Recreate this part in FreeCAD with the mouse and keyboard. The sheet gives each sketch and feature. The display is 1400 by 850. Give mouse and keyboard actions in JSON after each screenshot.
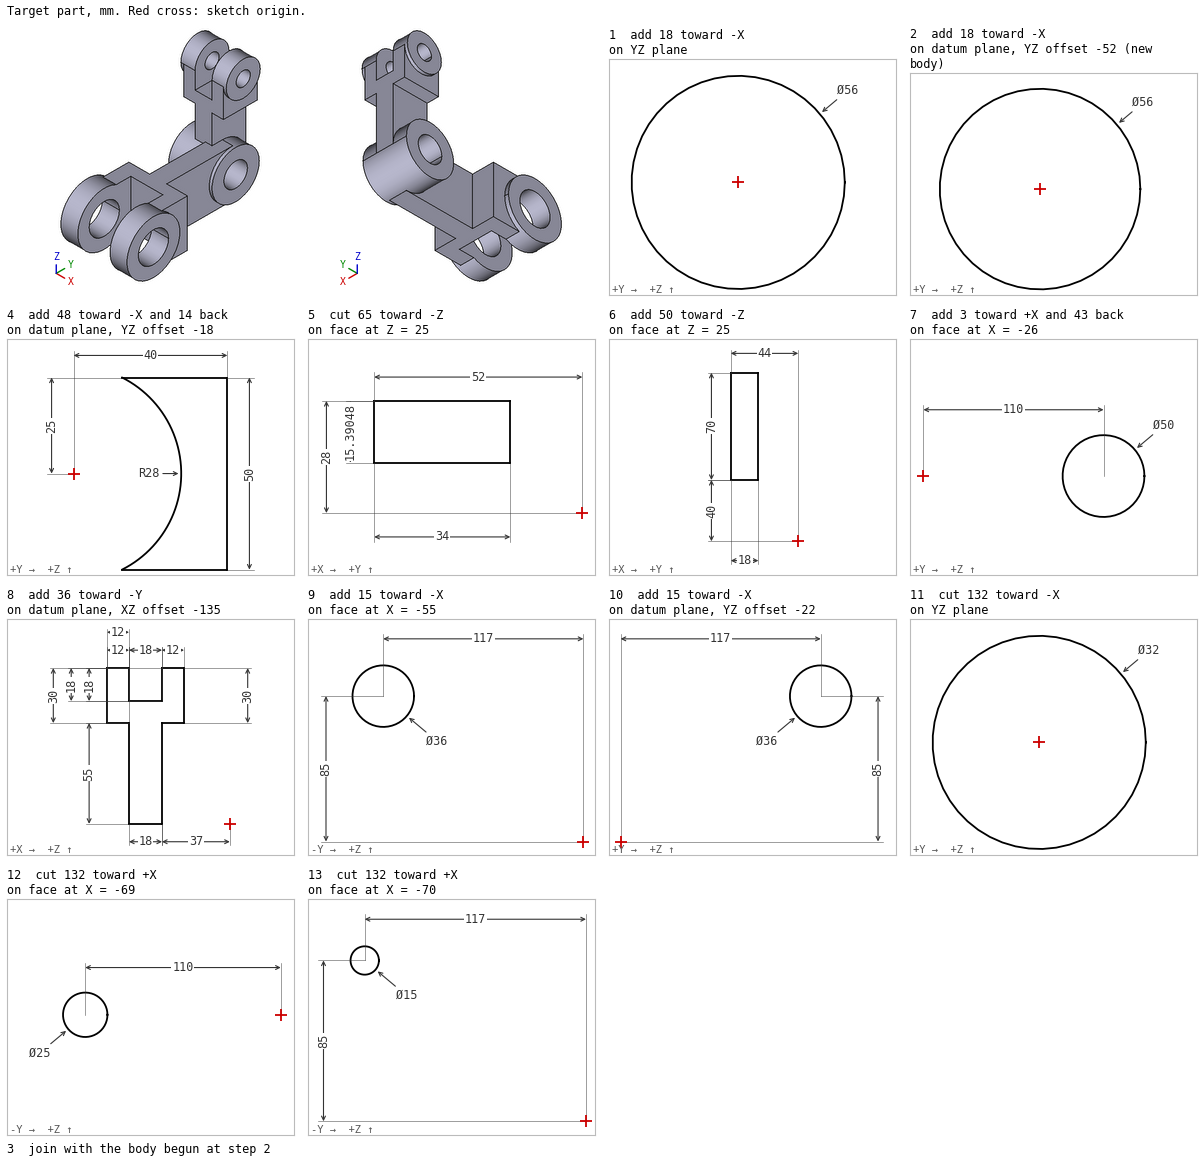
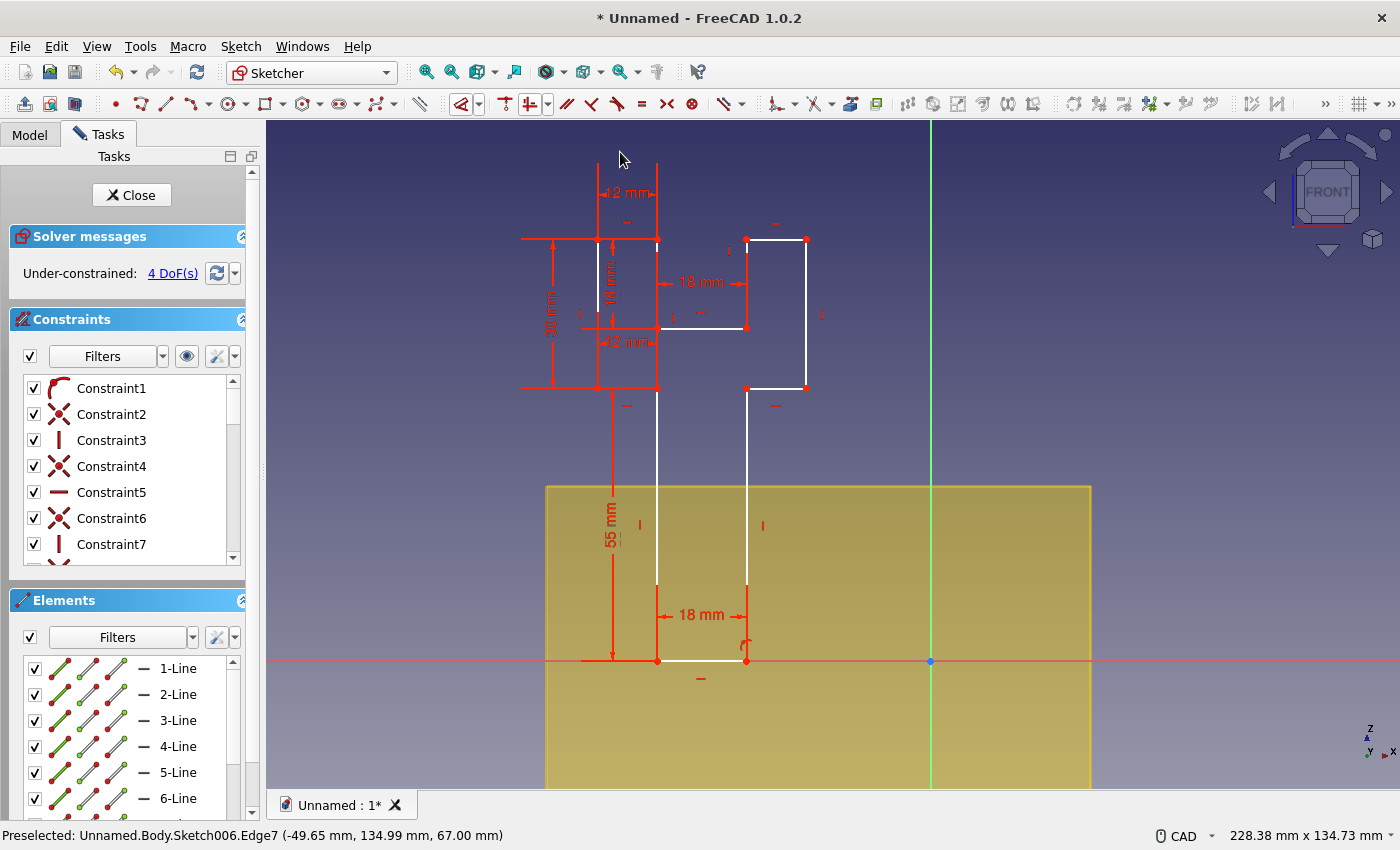
{"action": "left_click", "coordinate": [747, 302]}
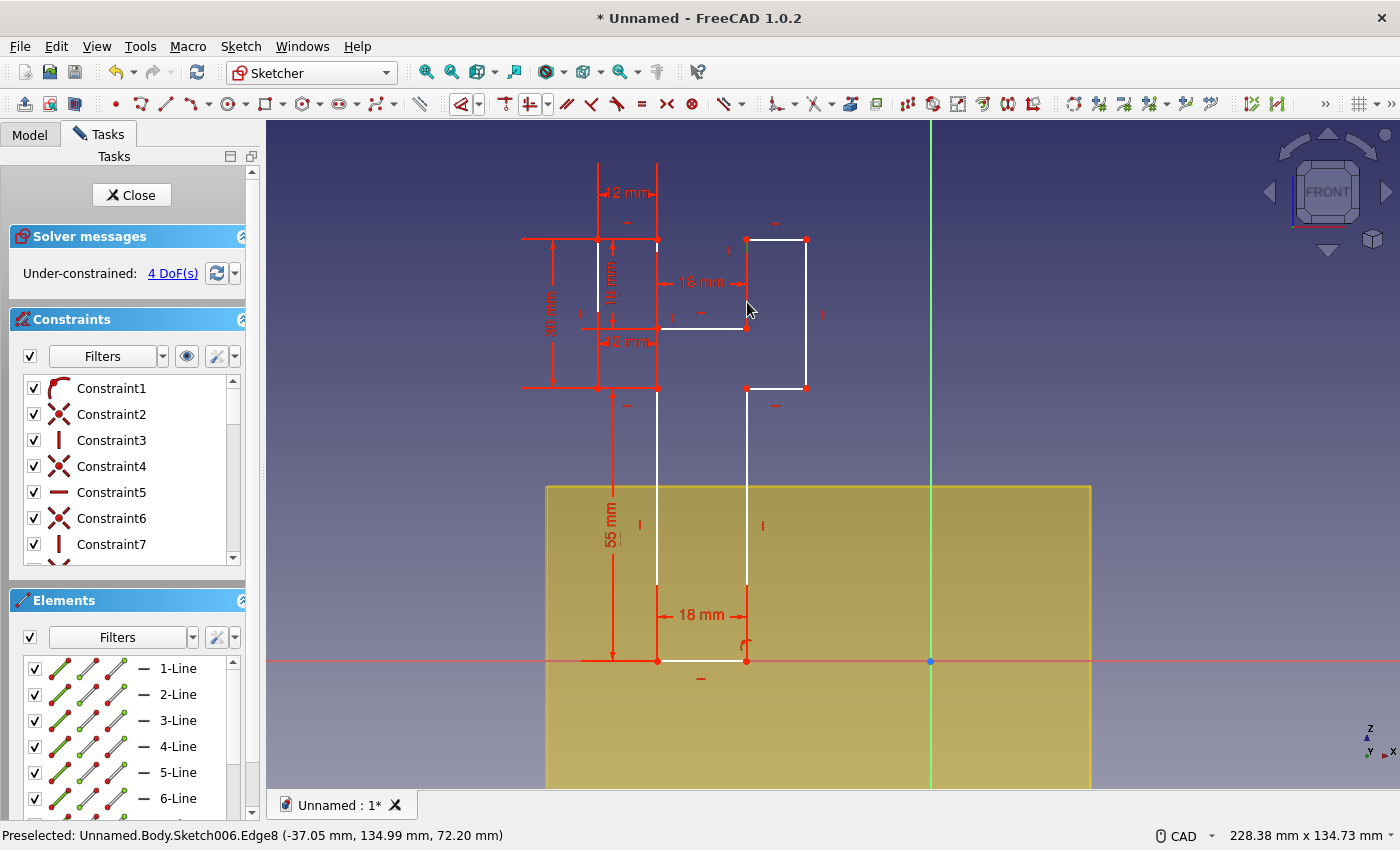
{"action": "key", "text": "i"}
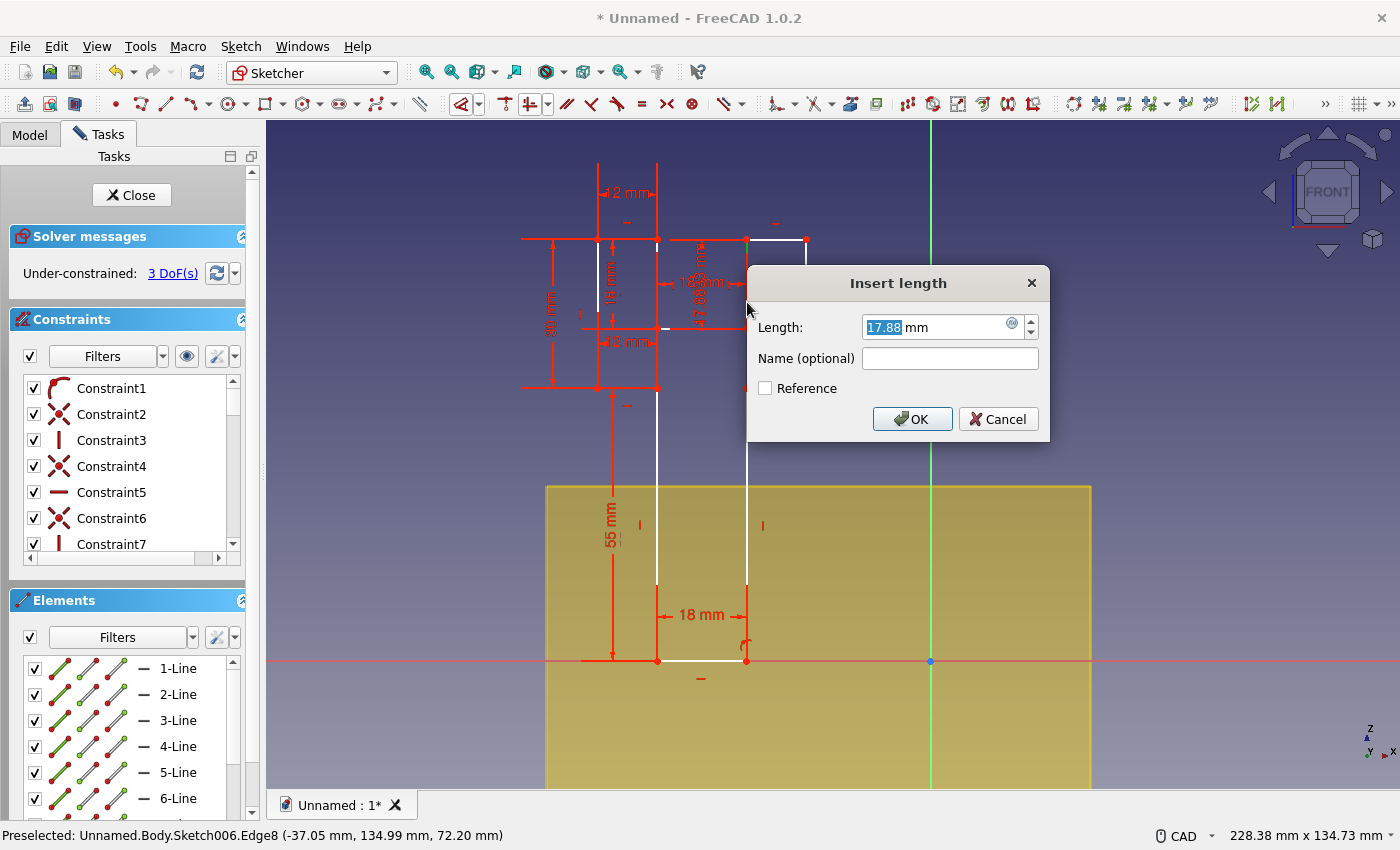
{"action": "type", "text": "18"}
{"action": "key", "text": "Return"}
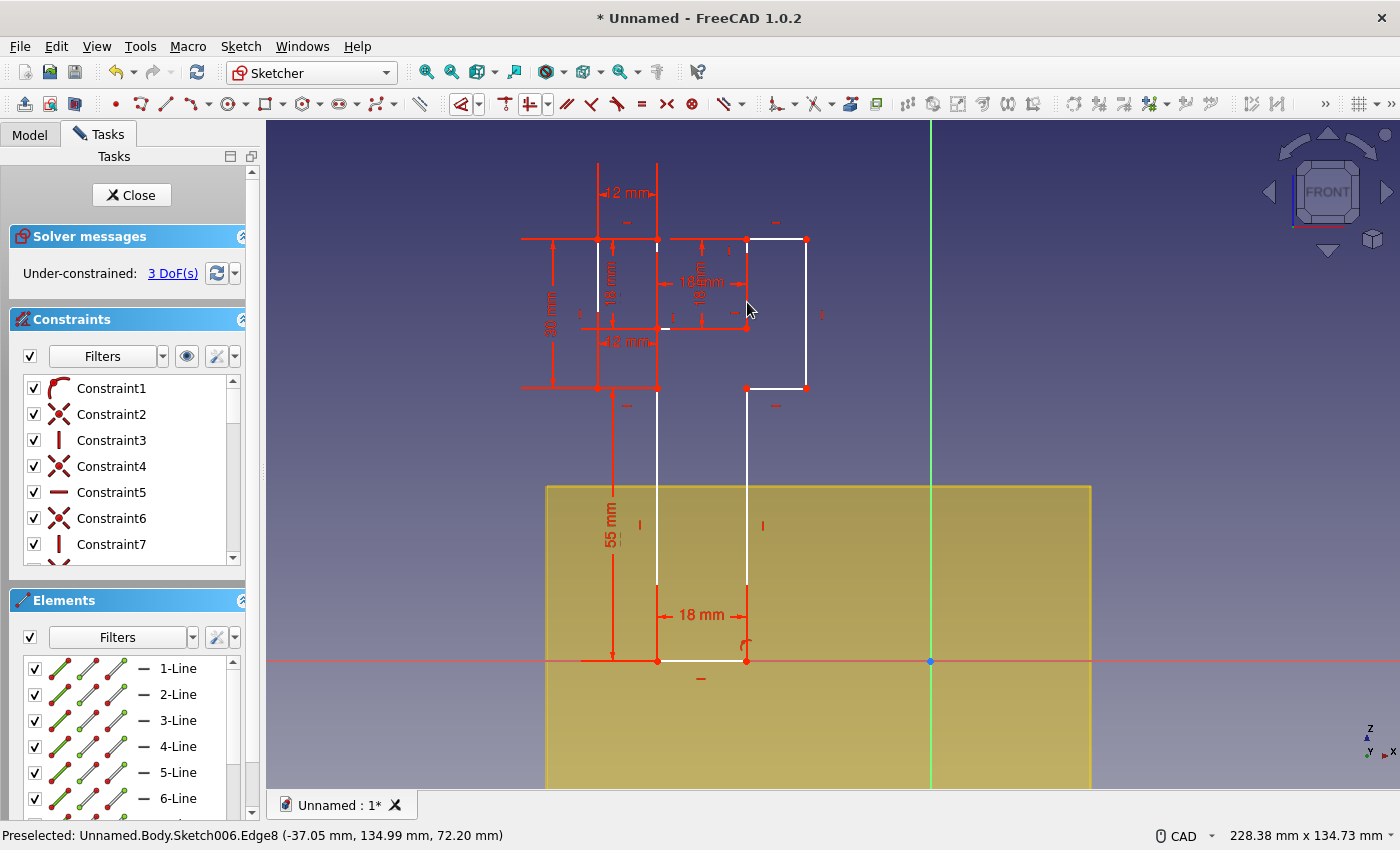
{"action": "left_click", "coordinate": [764, 239]}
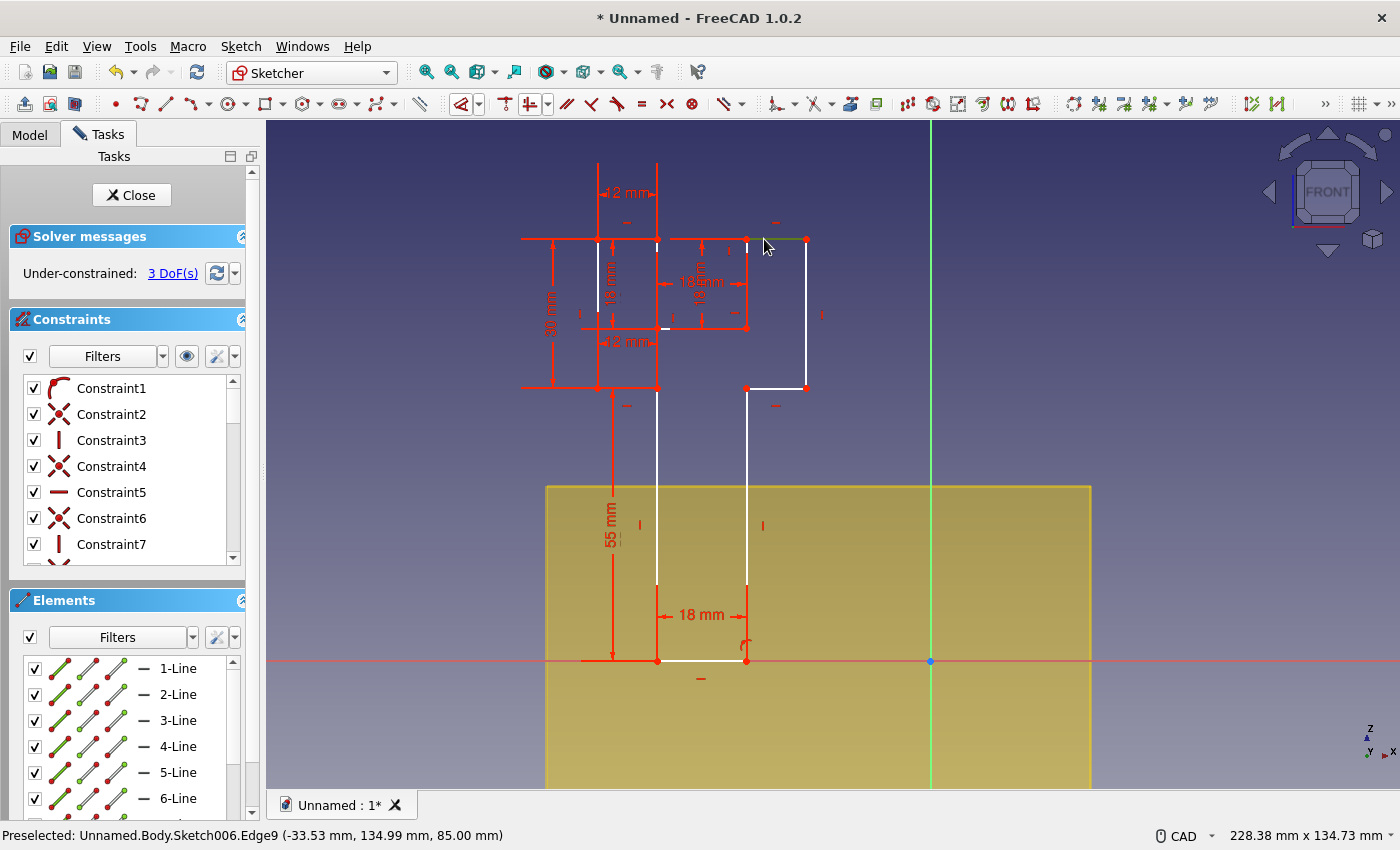
{"action": "key", "text": "l"}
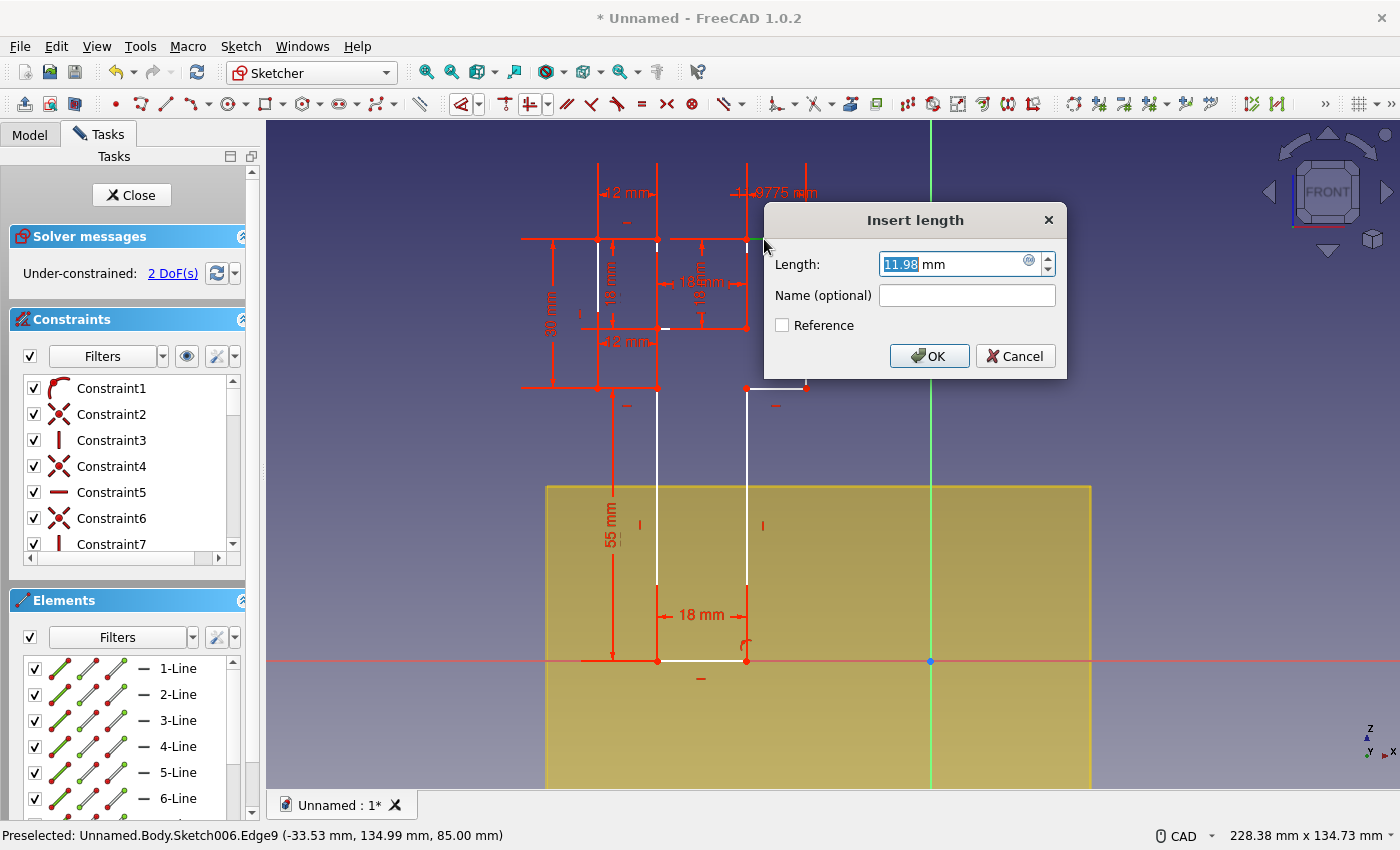
{"action": "type", "text": "12"}
{"action": "key", "text": "Return"}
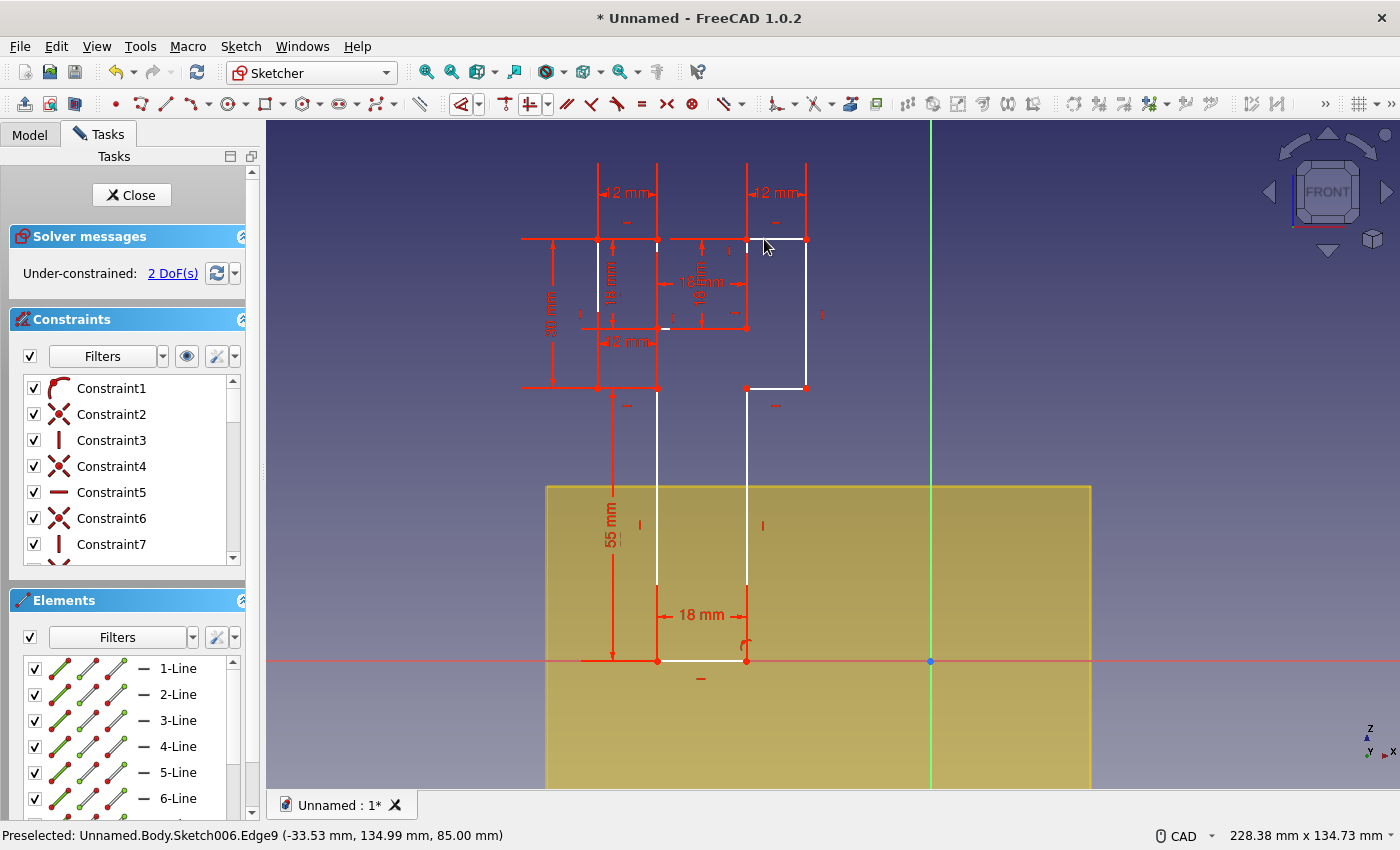
{"action": "left_click", "coordinate": [806, 284]}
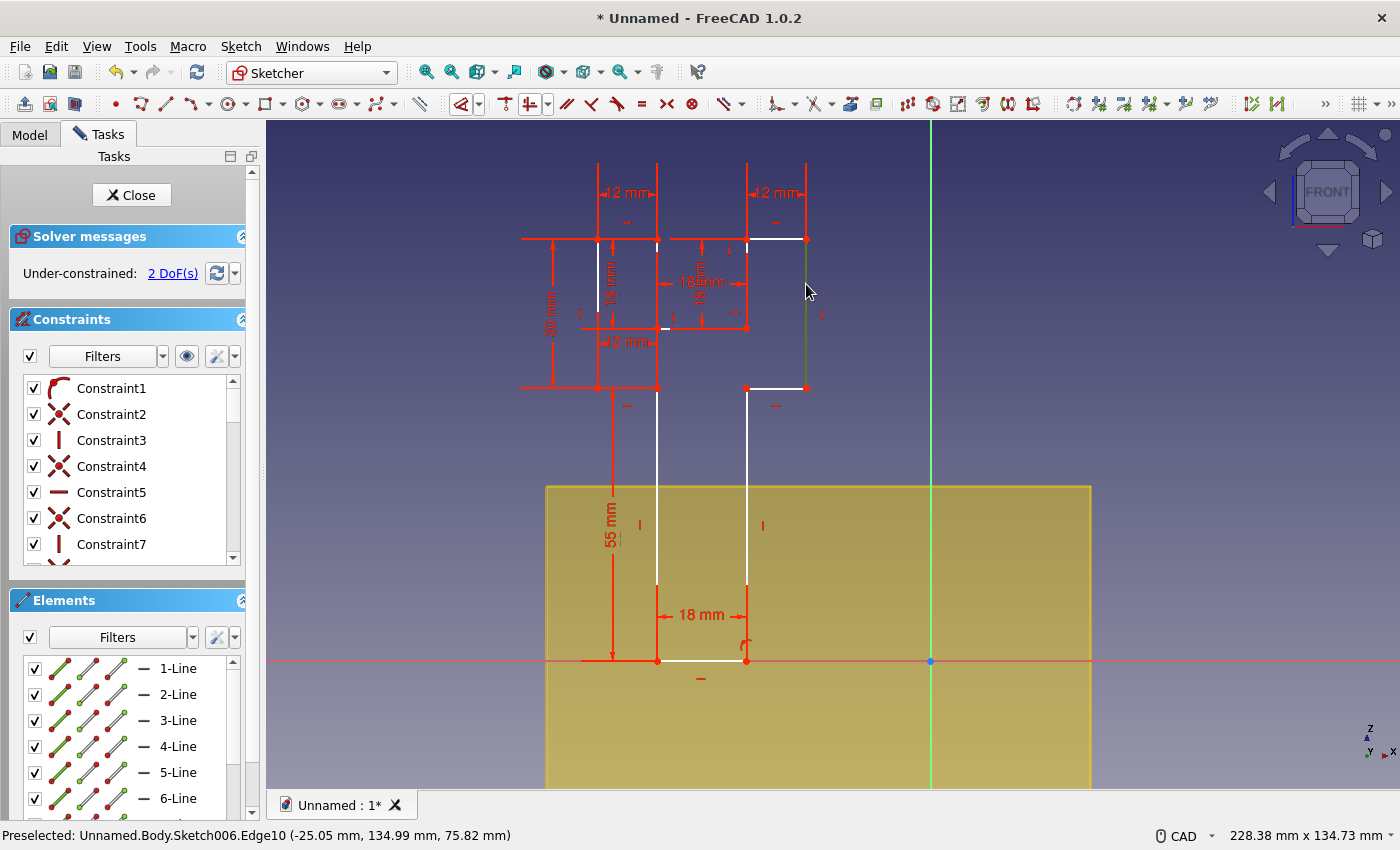
{"action": "key", "text": "i"}